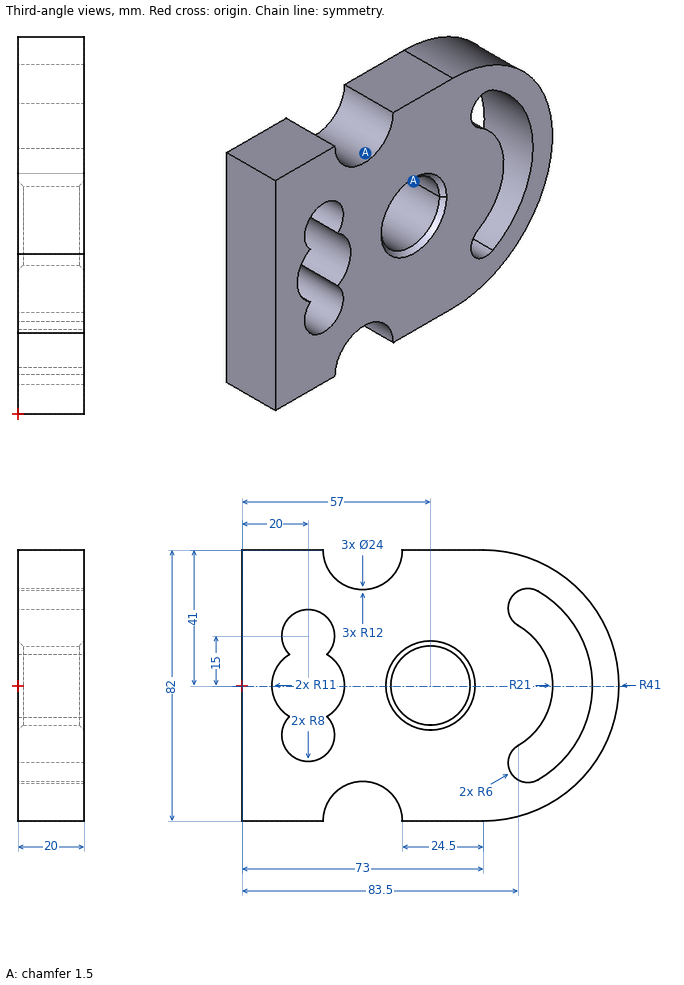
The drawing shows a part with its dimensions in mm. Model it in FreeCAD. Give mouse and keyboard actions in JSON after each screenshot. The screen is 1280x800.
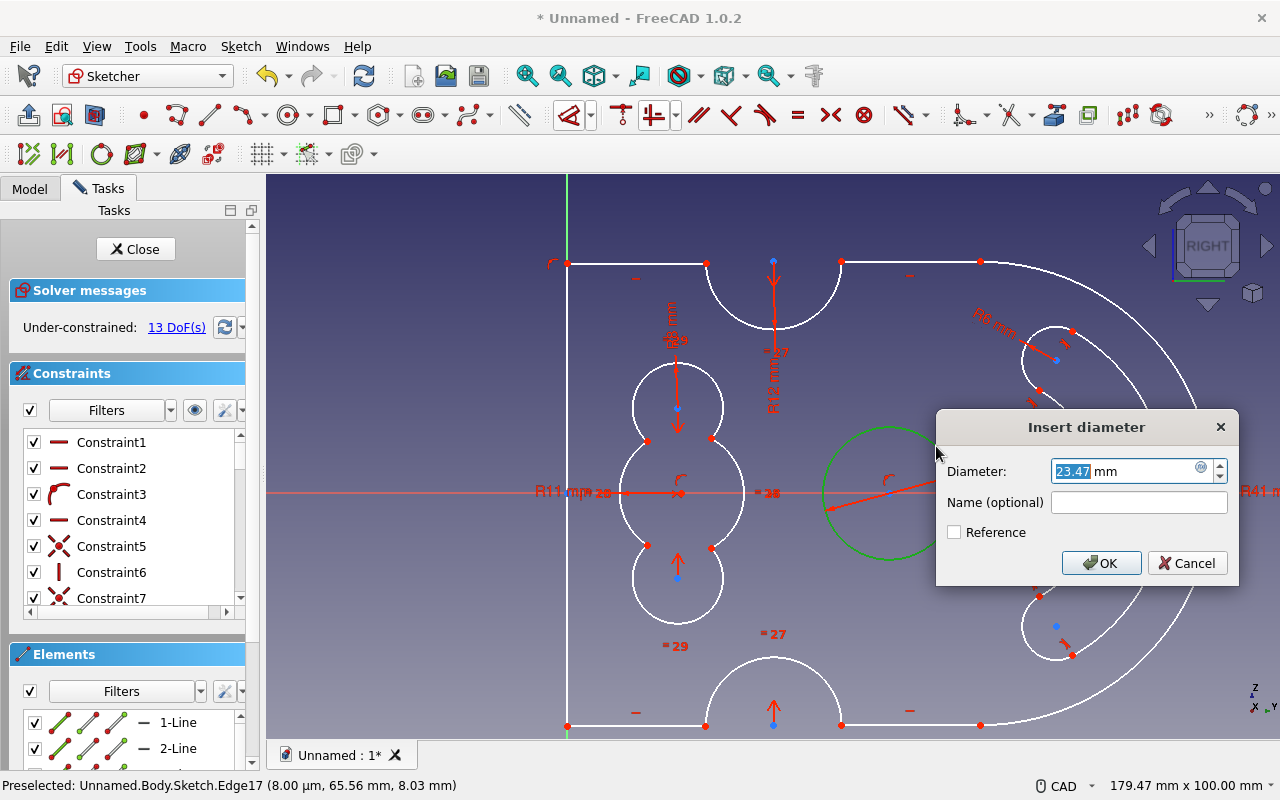
{"action": "type", "text": "24"}
{"action": "key", "text": "Return"}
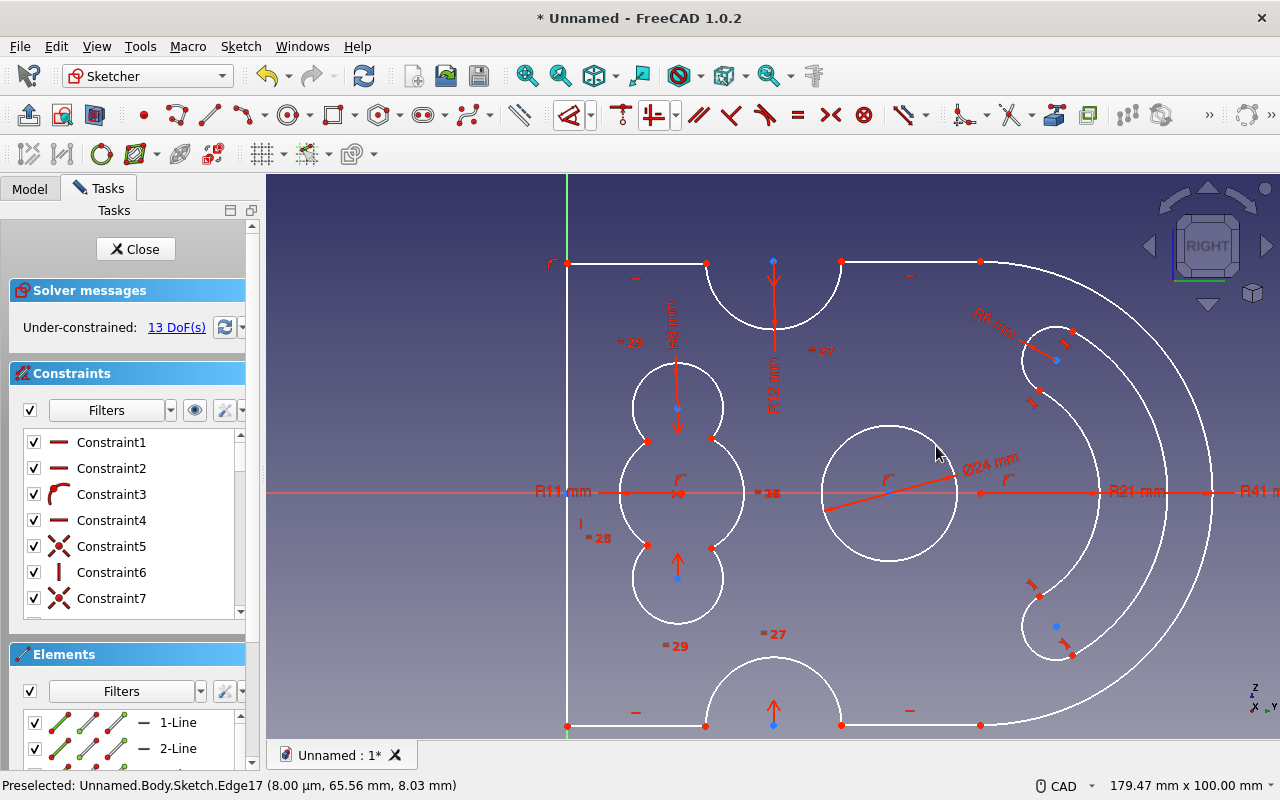
{"action": "left_click", "coordinate": [567, 403]}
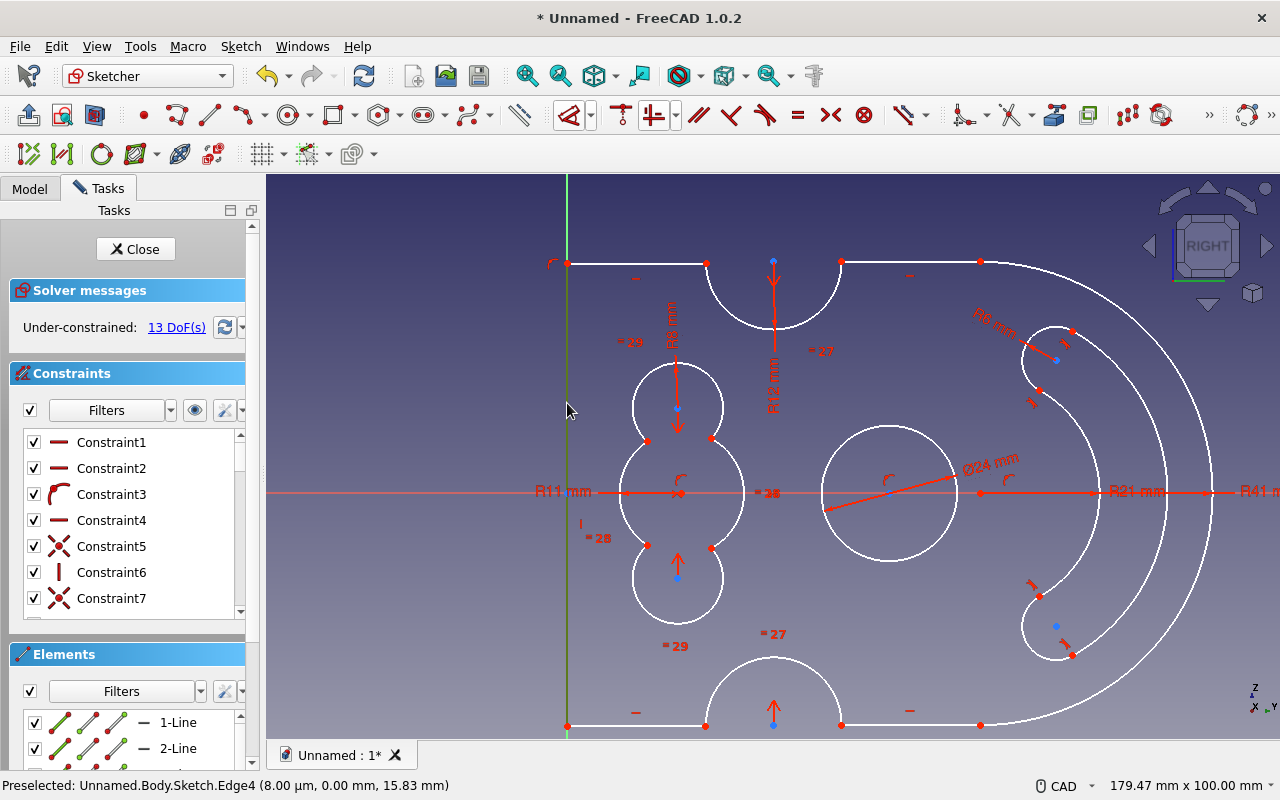
{"action": "key", "text": "i"}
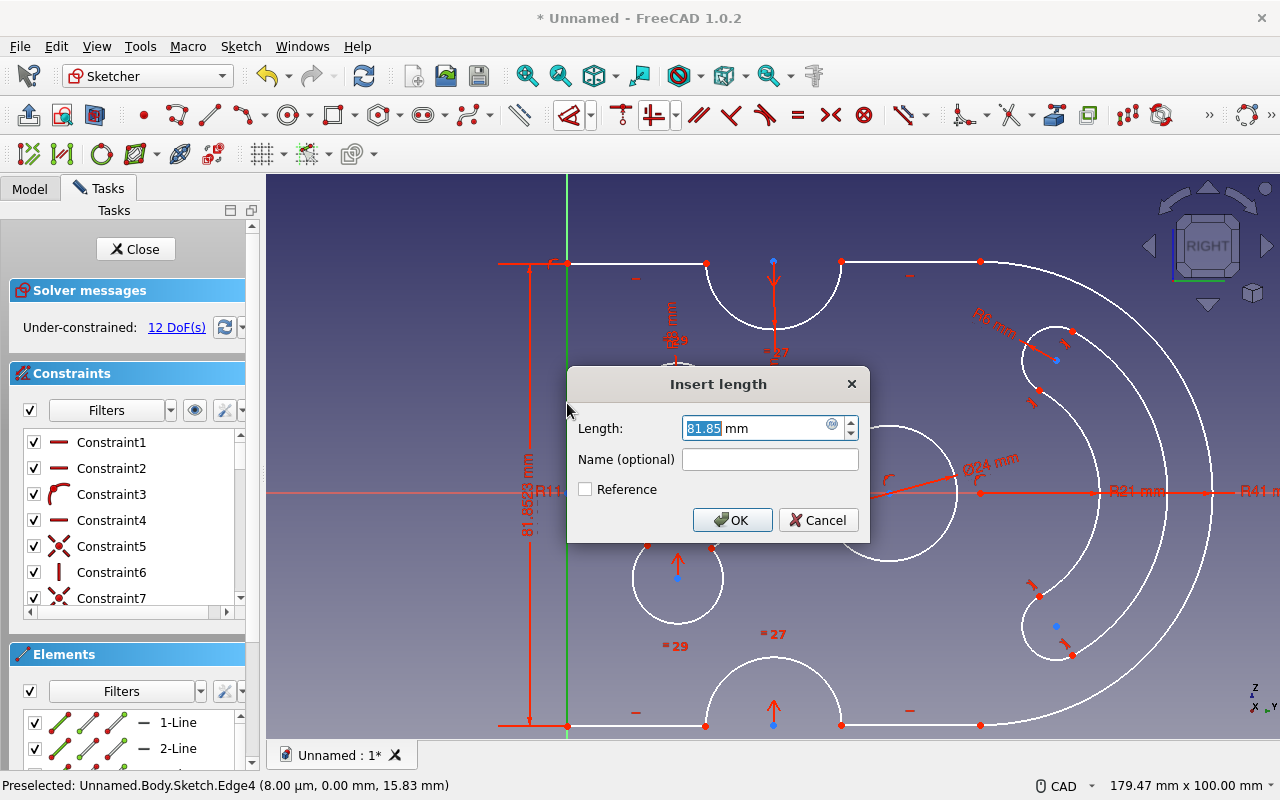
{"action": "type", "text": "82"}
{"action": "key", "text": "Return"}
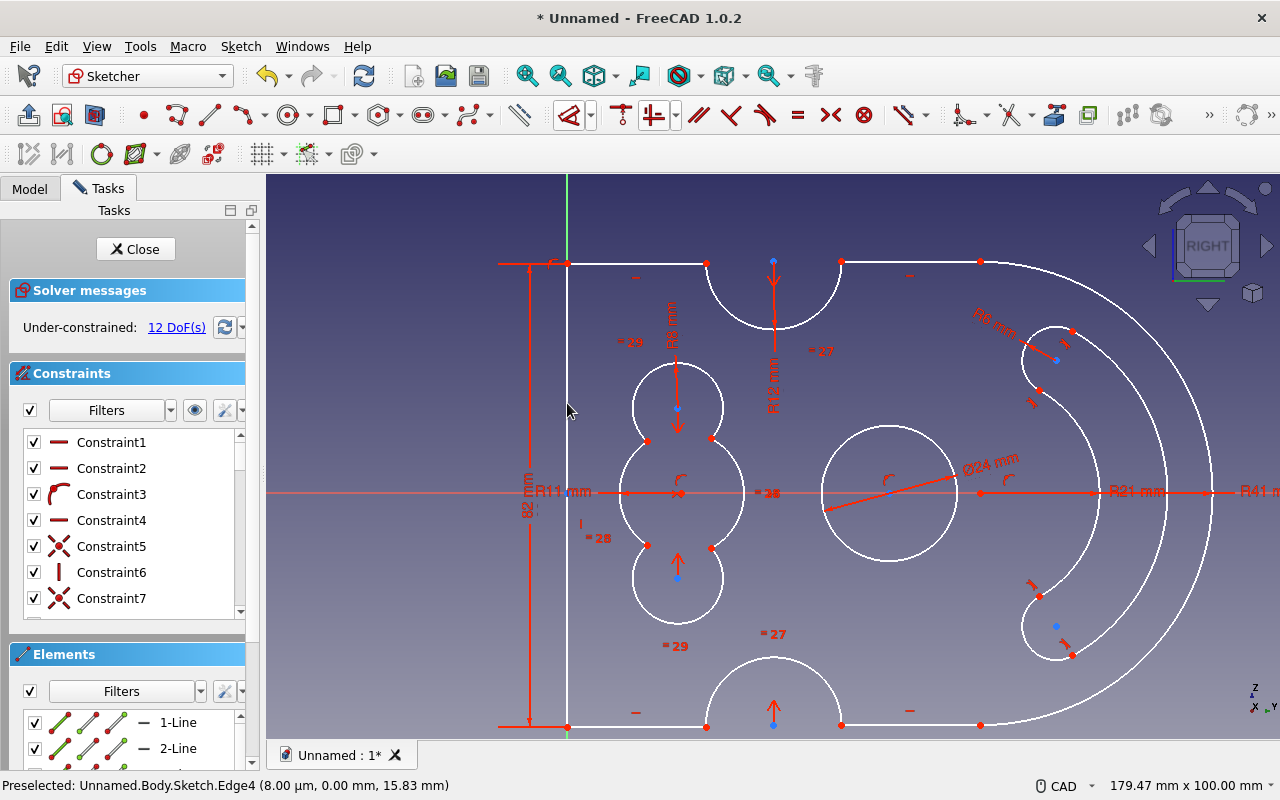
{"action": "left_click", "coordinate": [889, 493]}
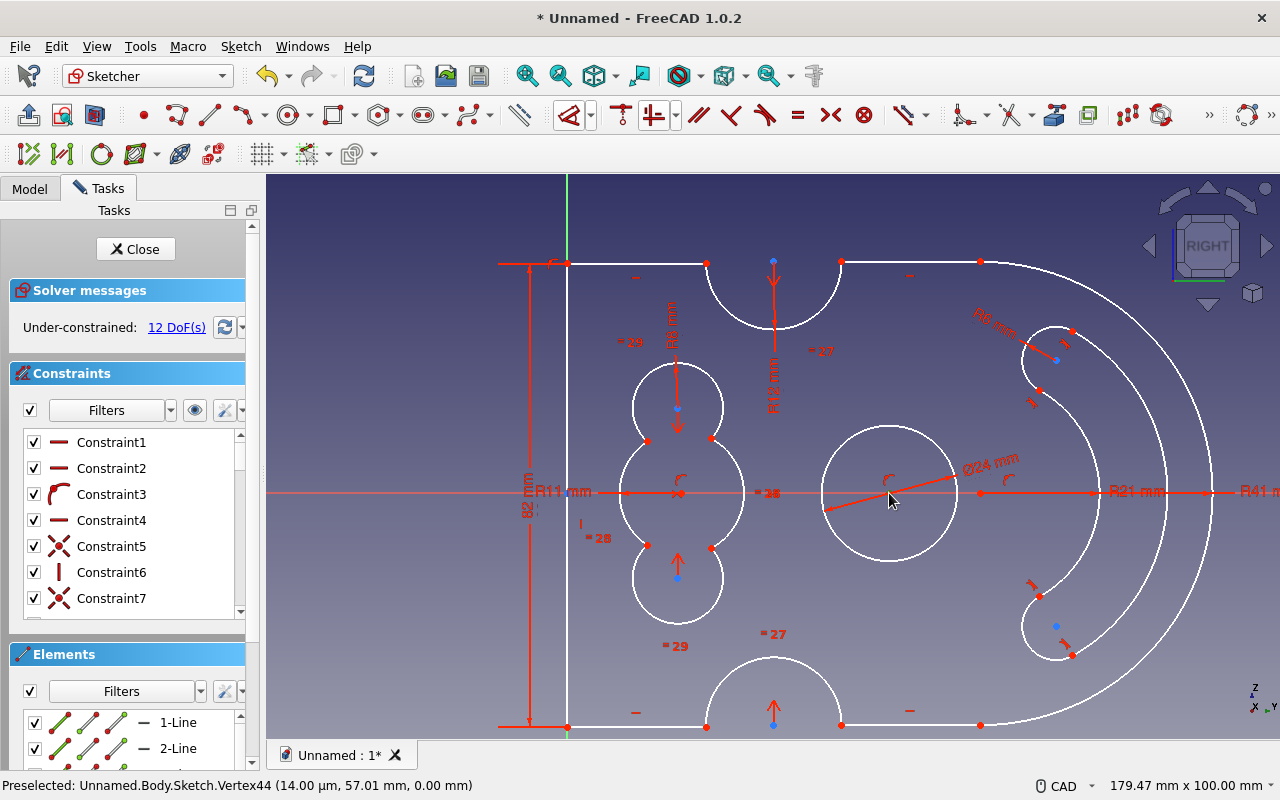
{"action": "key", "text": "l"}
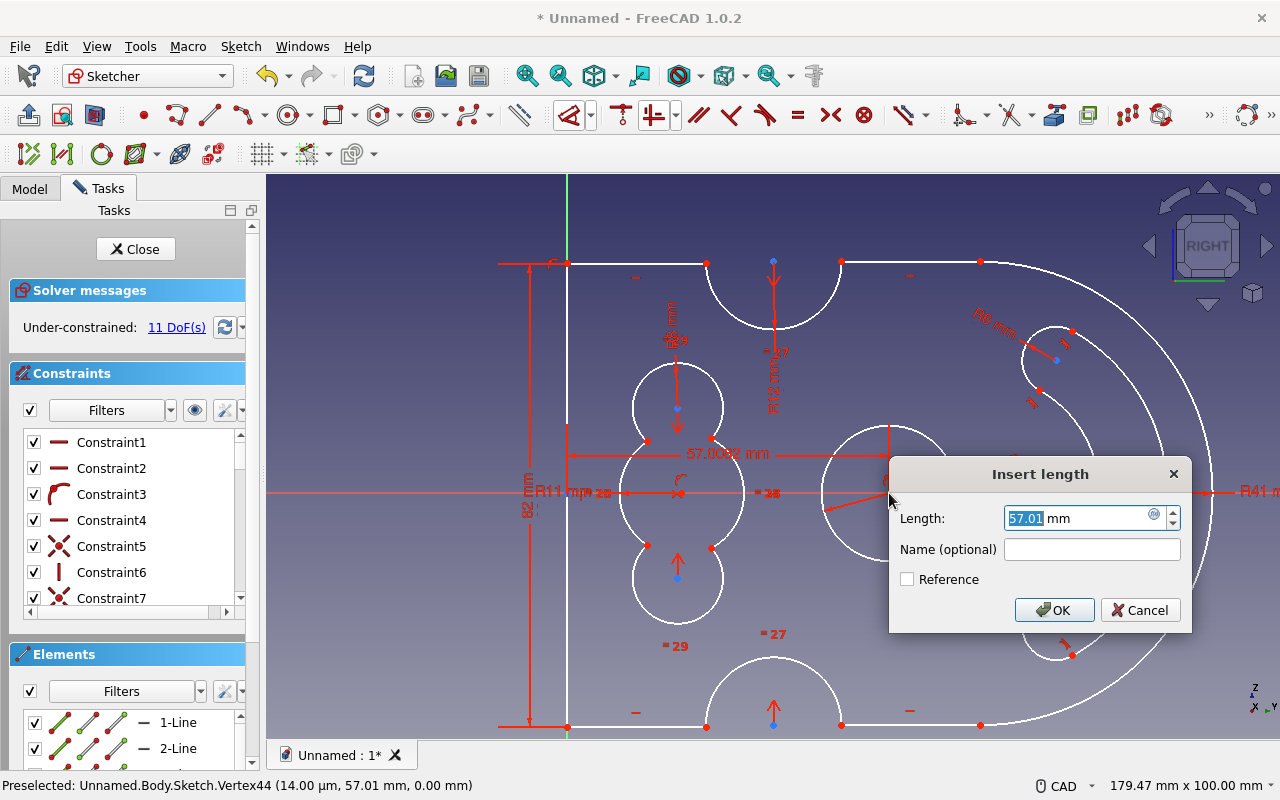
{"action": "type", "text": "57"}
{"action": "key", "text": "Return"}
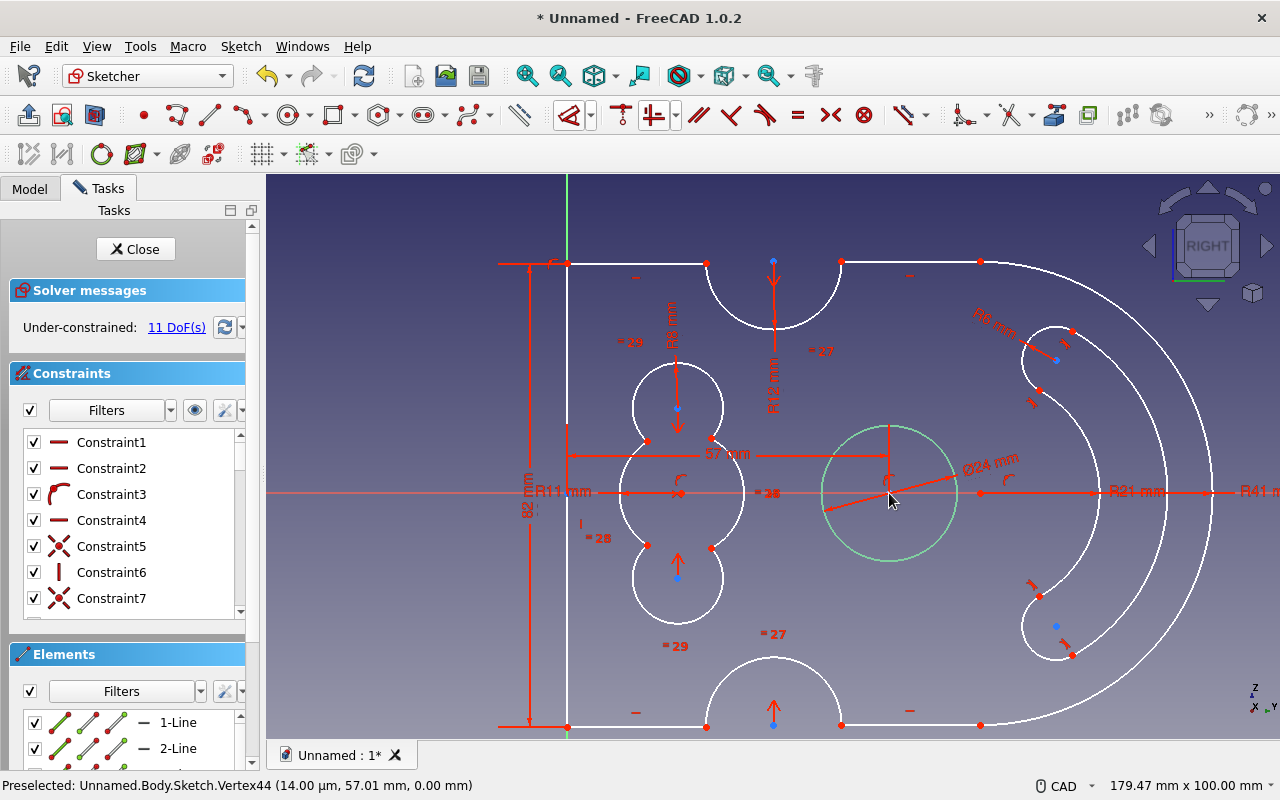
{"action": "scroll", "coordinate": [294, 290], "scroll_direction": "down", "scroll_amount": 1}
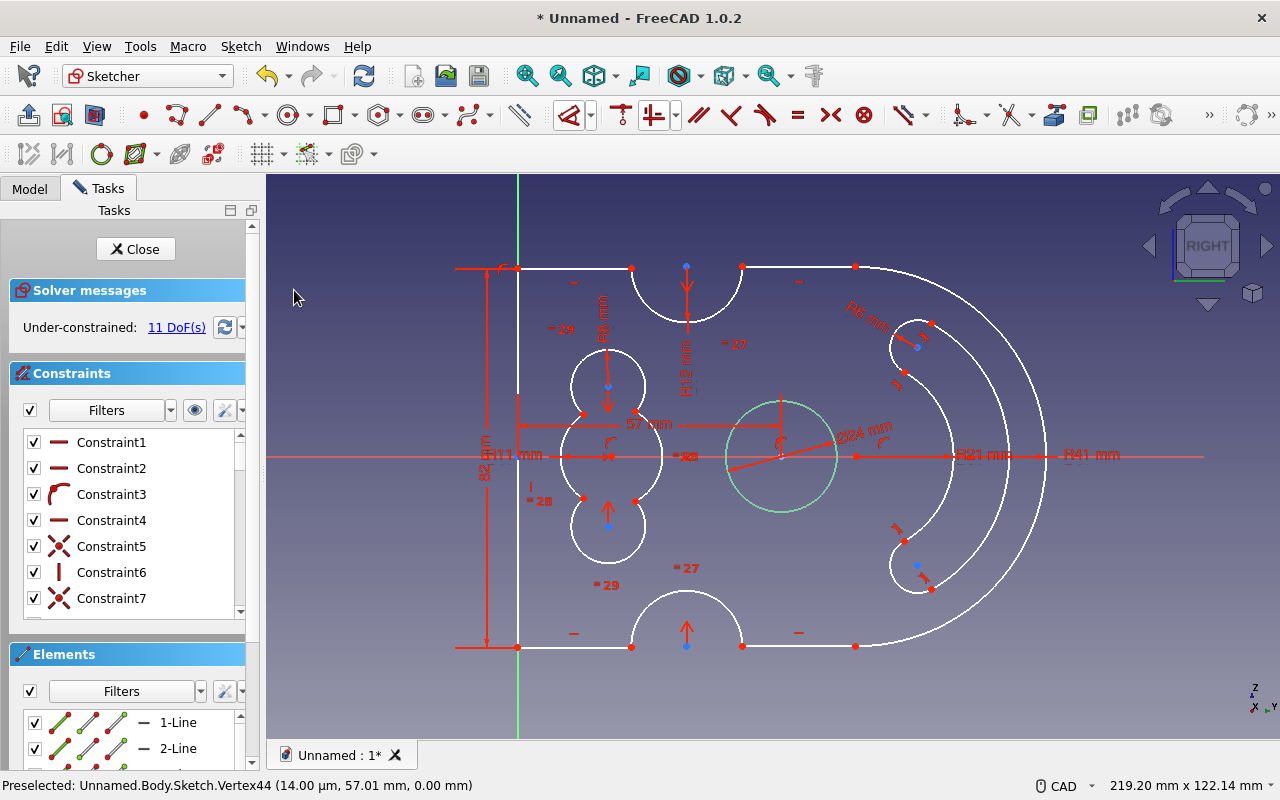
{"action": "left_click", "coordinate": [856, 646]}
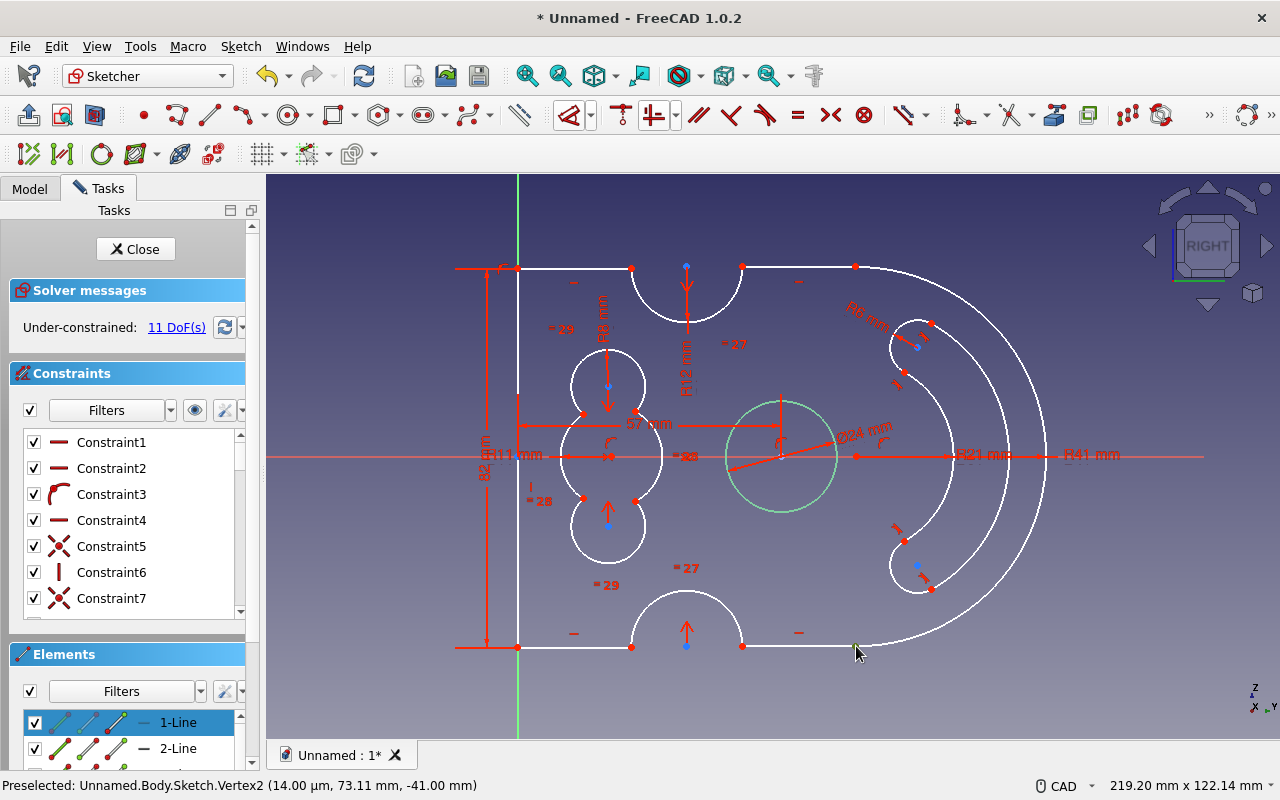
{"action": "key", "text": "l"}